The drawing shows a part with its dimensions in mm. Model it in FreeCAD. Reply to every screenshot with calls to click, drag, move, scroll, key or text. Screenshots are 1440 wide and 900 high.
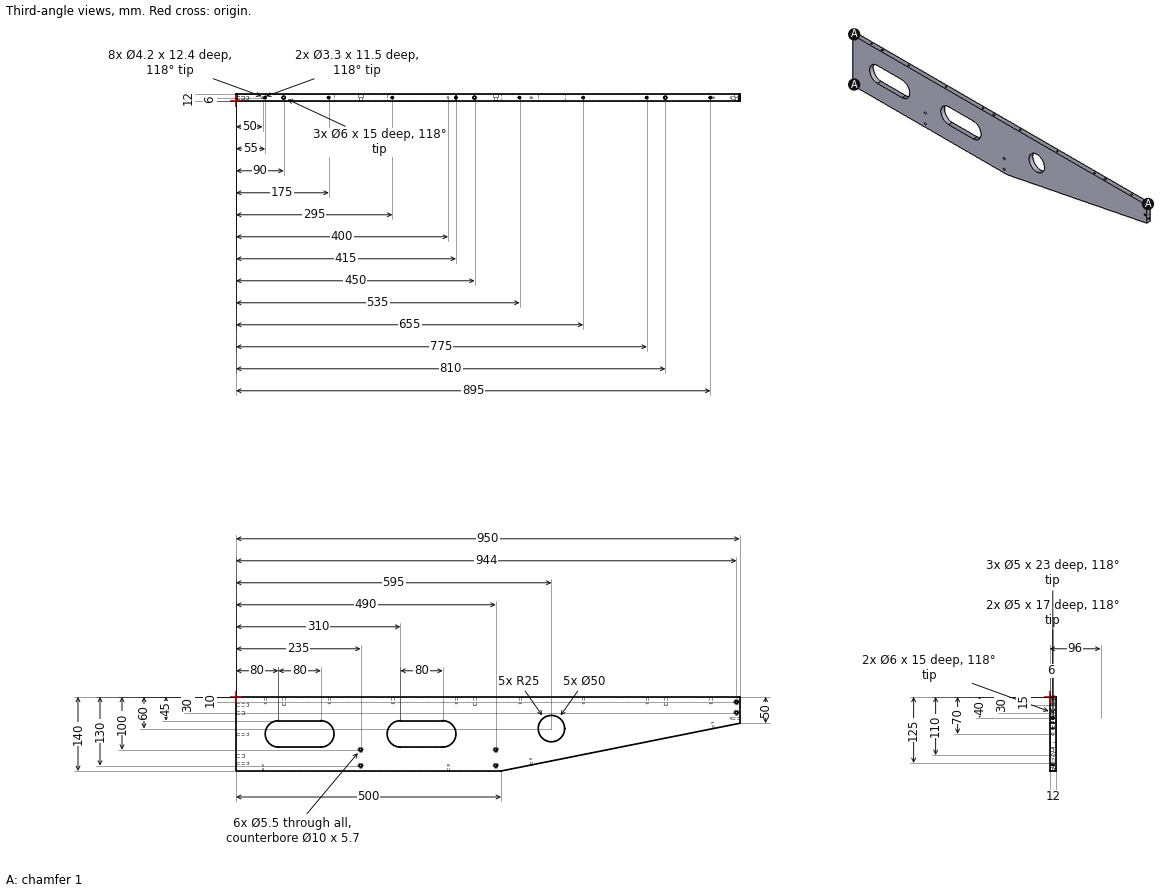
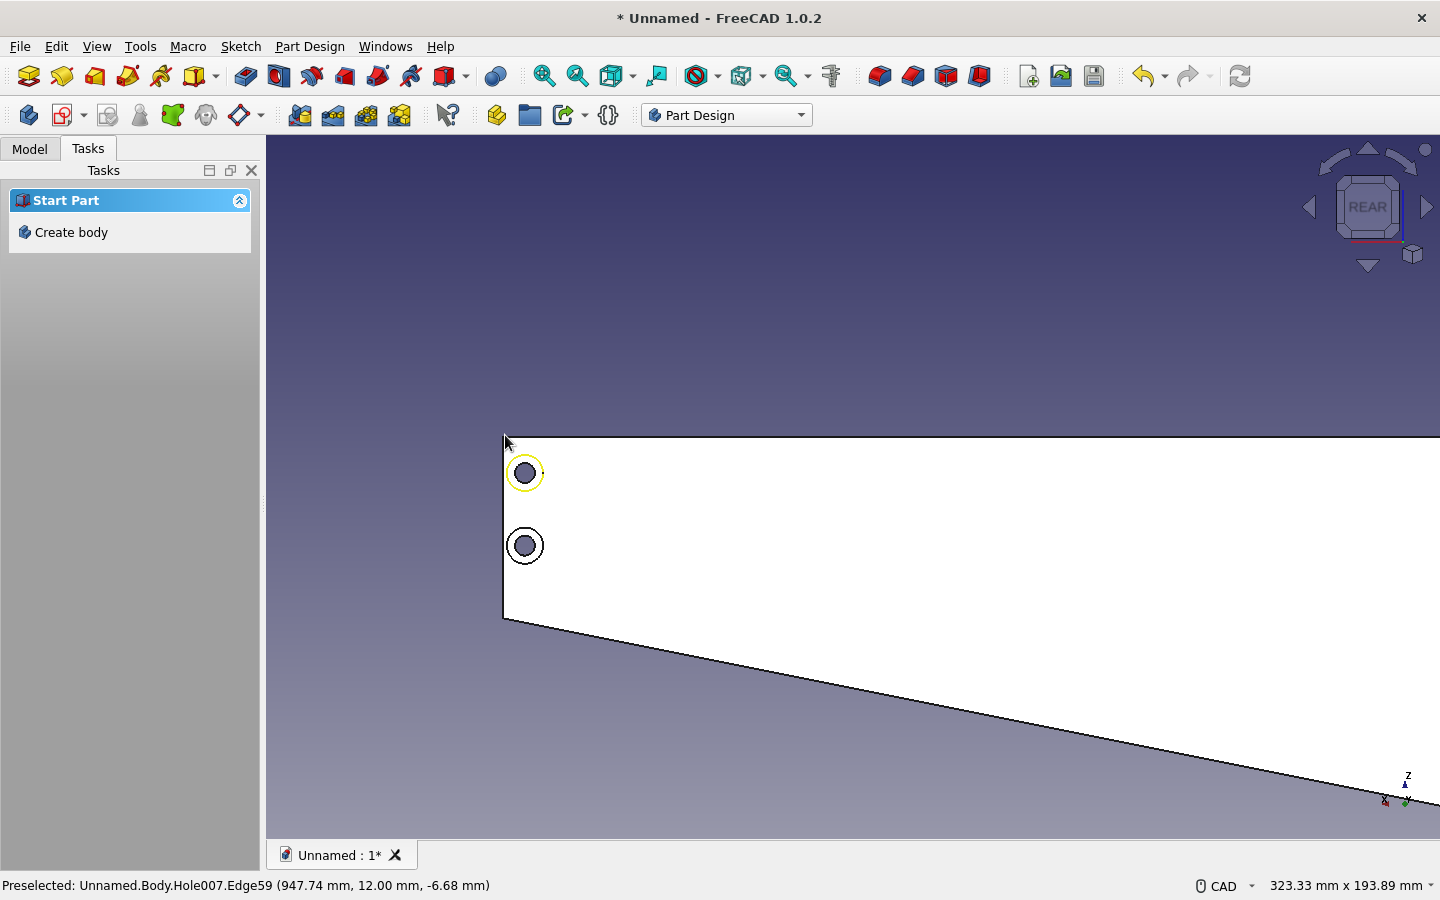
key(v)
key(f)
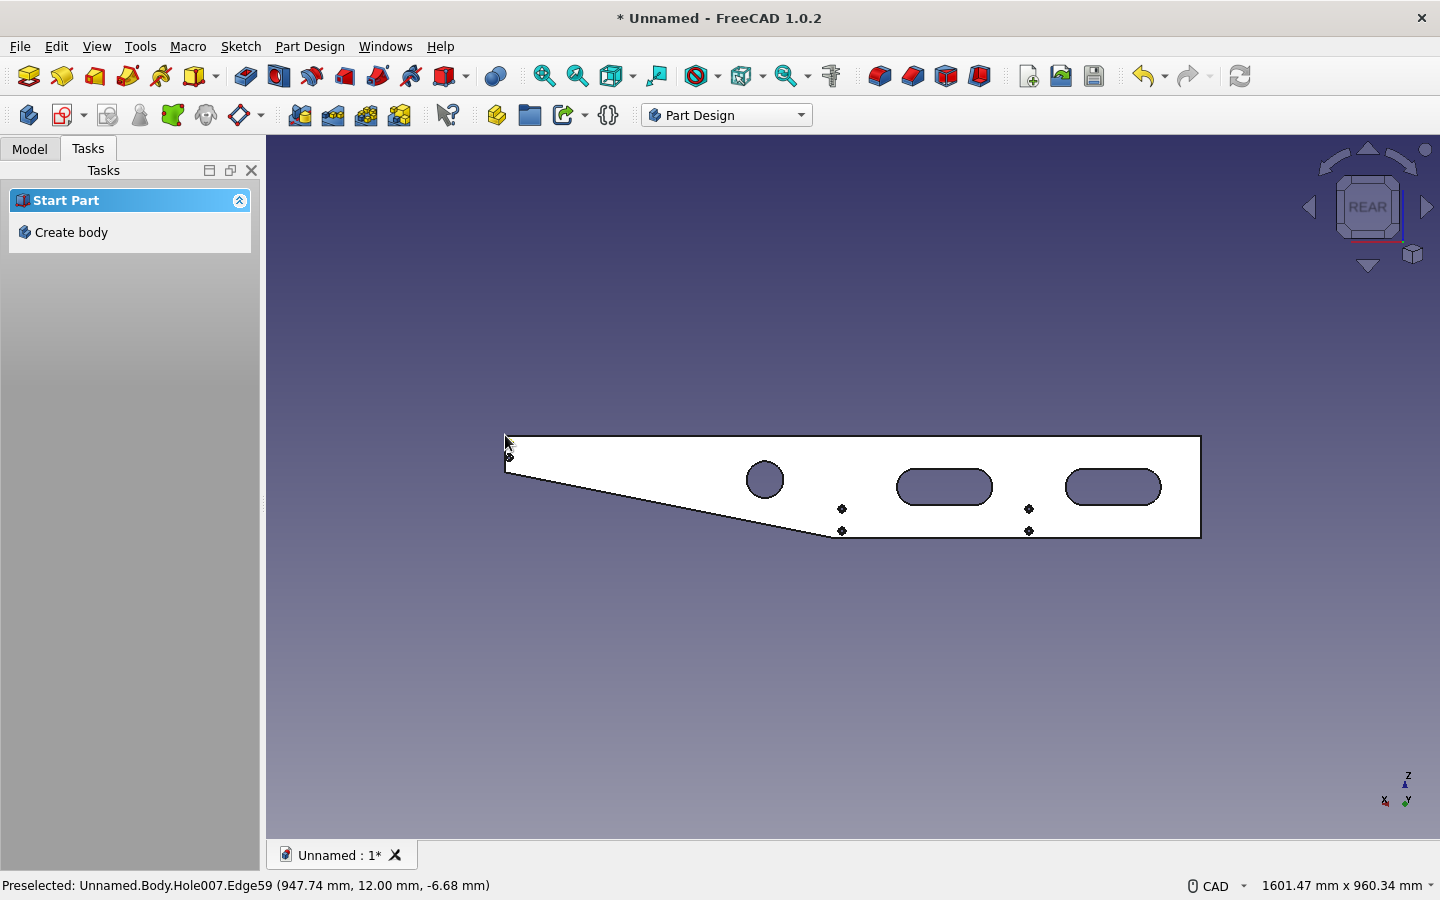
key(0)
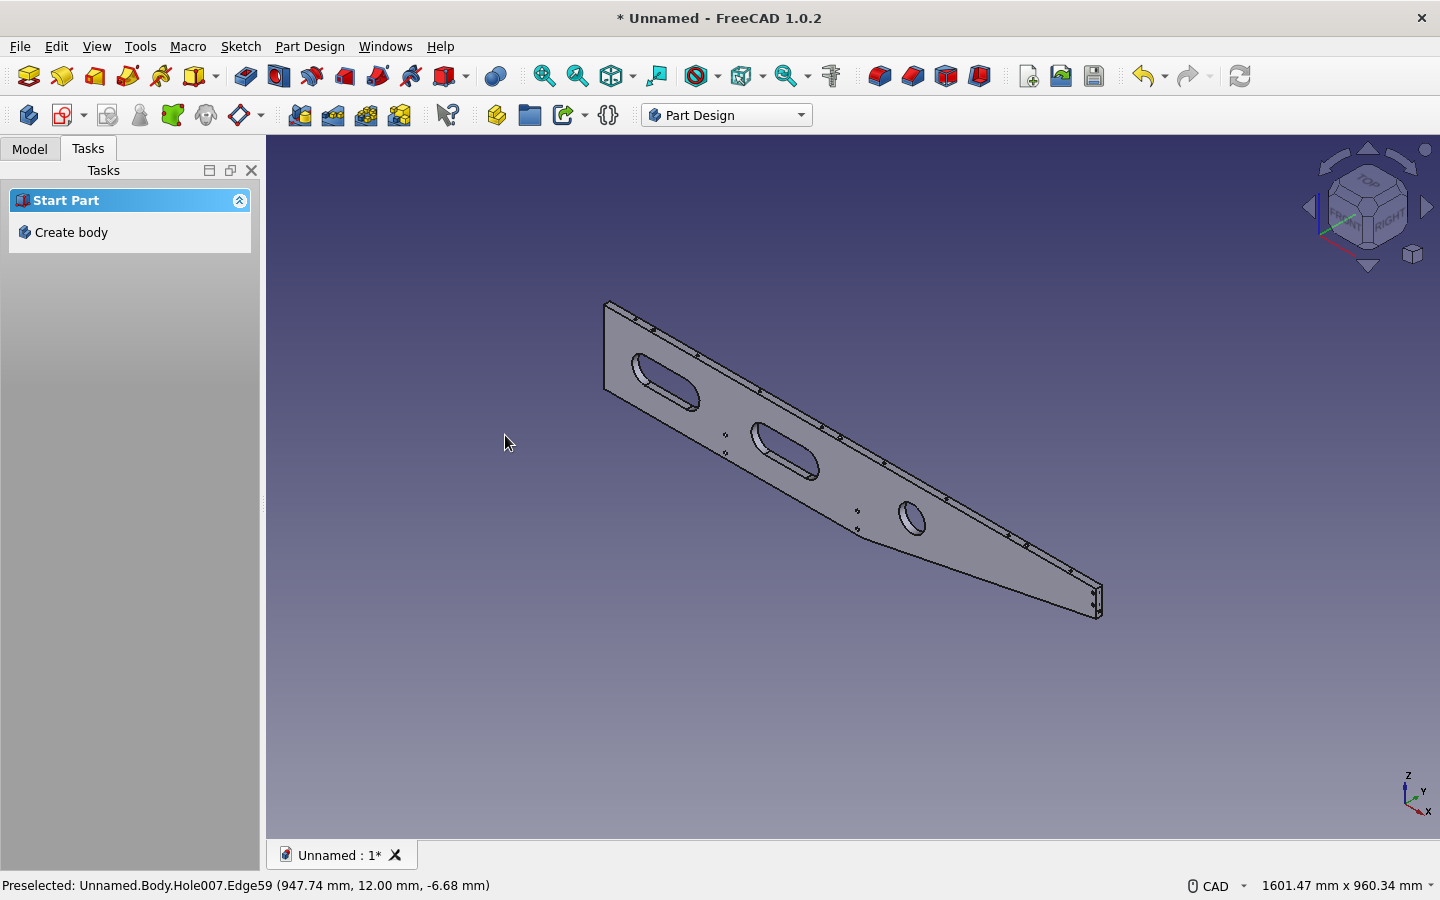
scroll(1099, 586, up, 8)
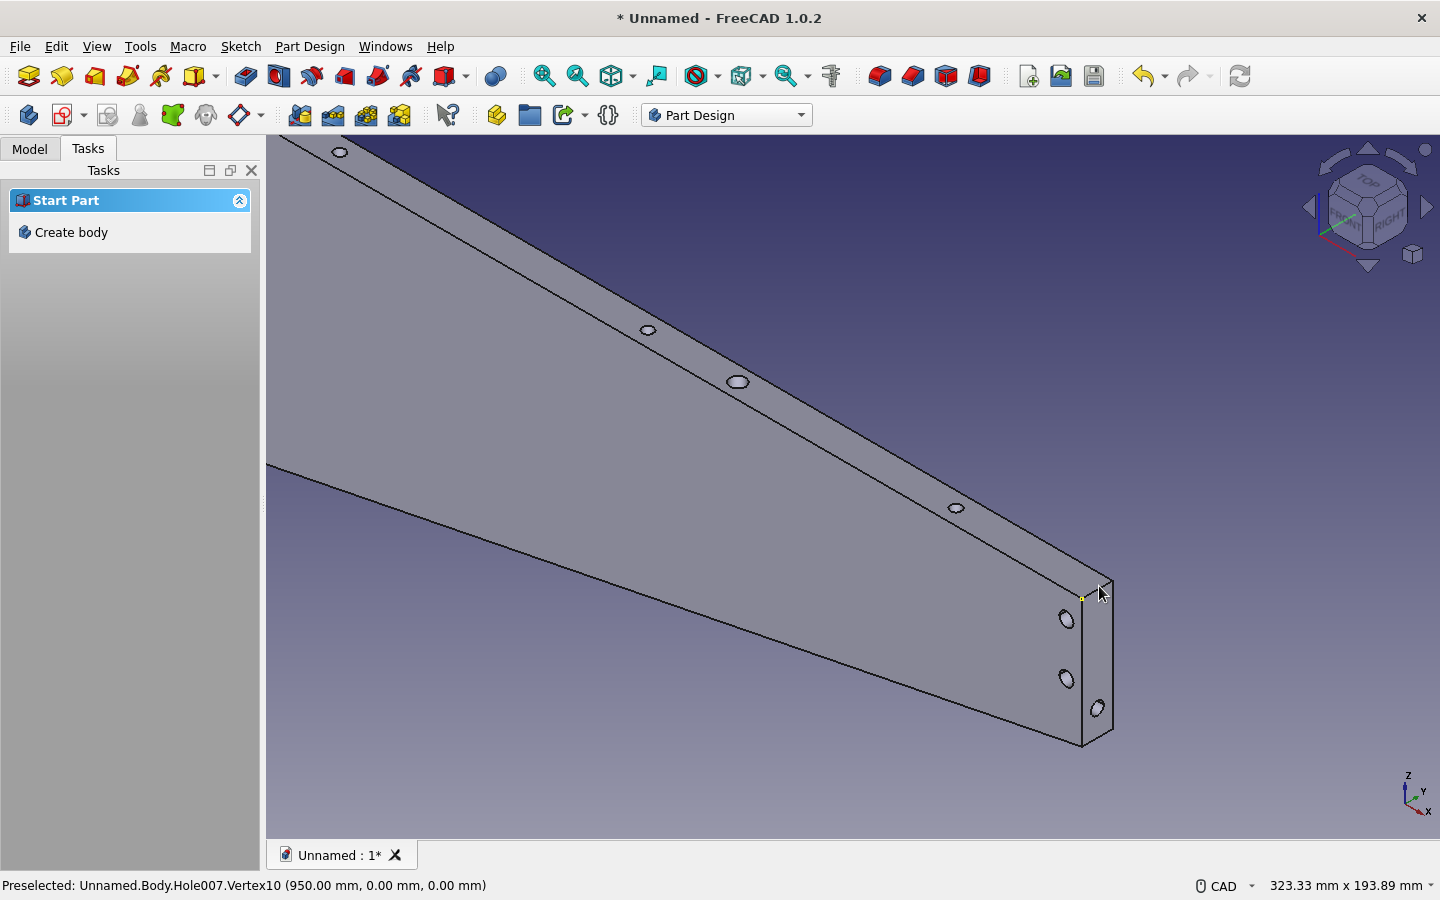
click(1097, 589)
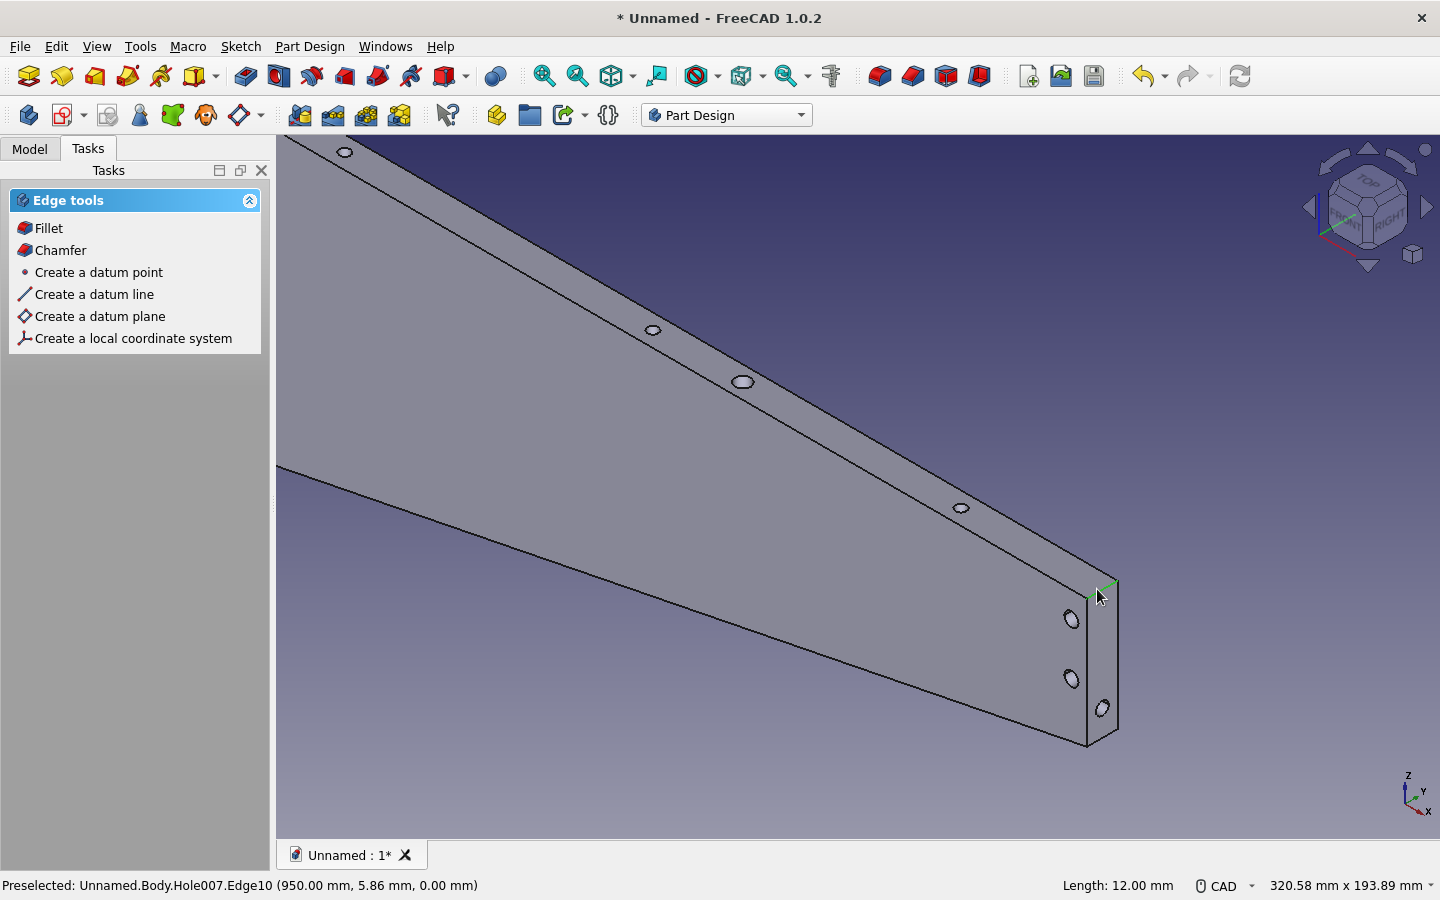
key(v)
key(f)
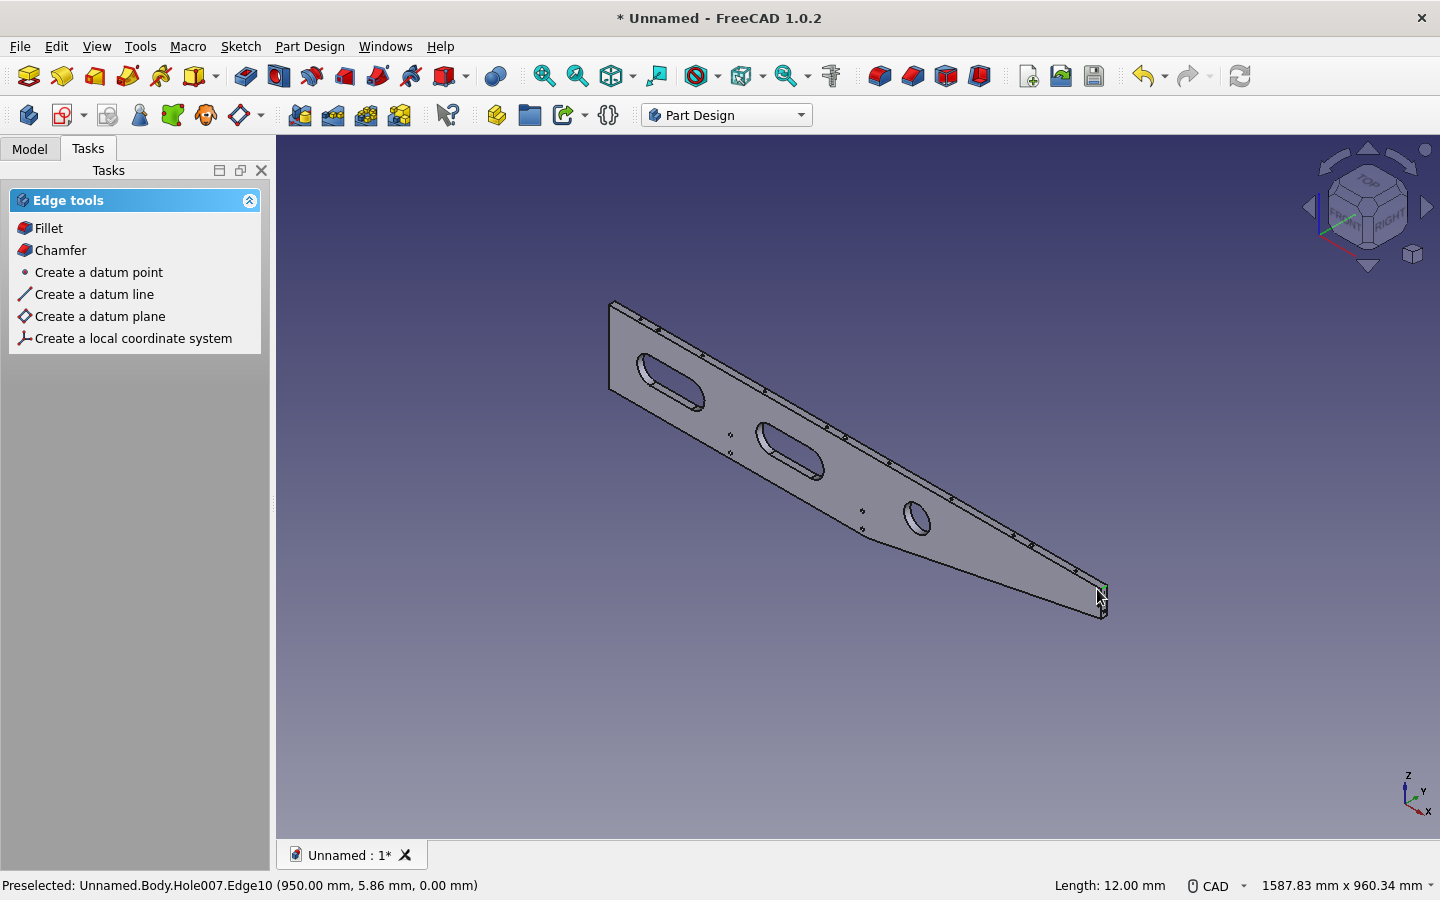
key(2)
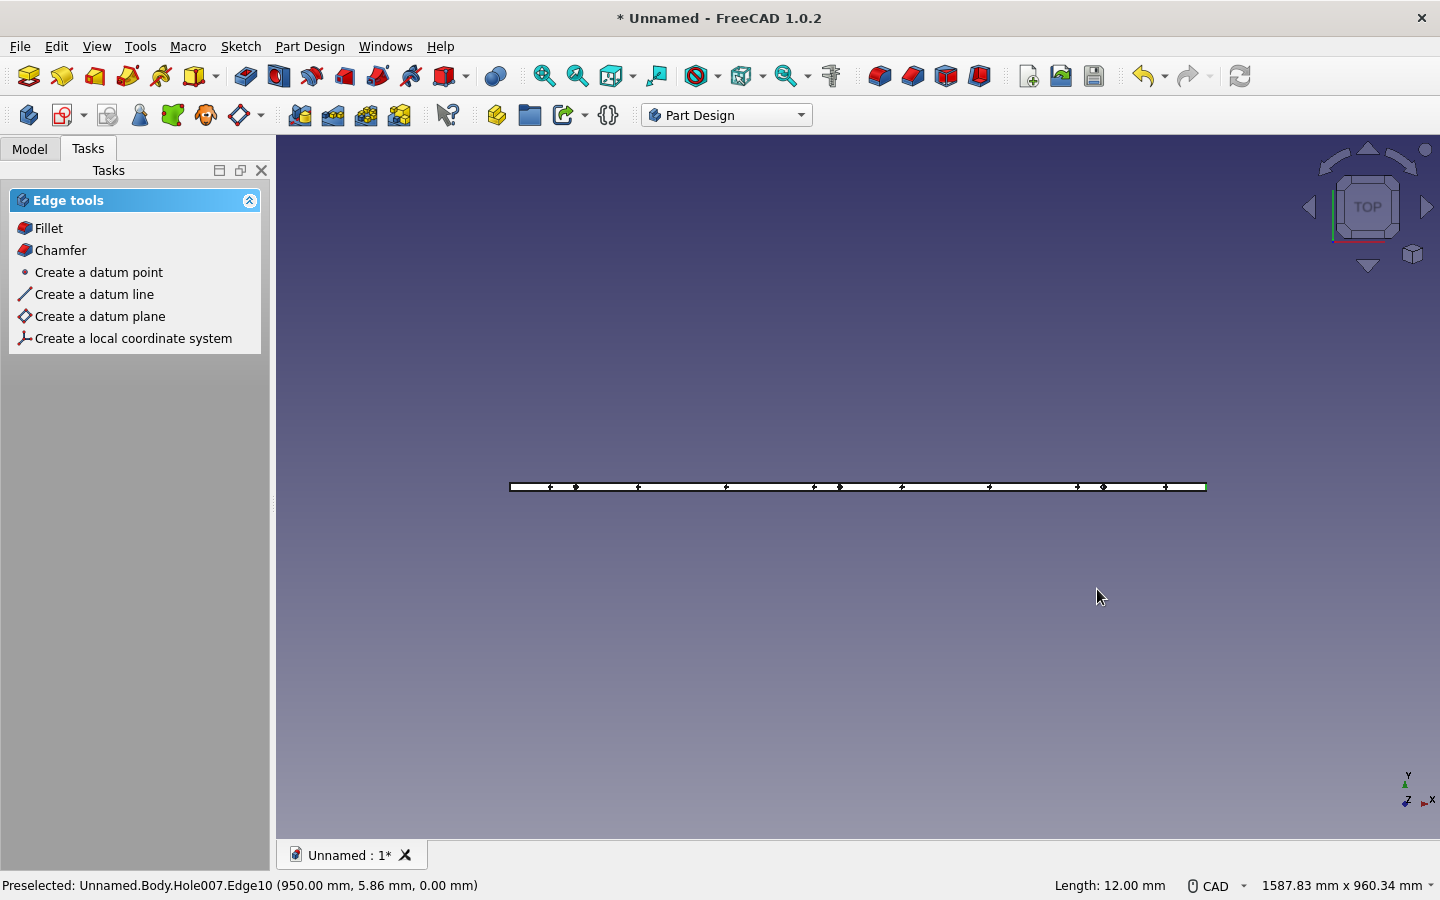
click(510, 488, ctrl)